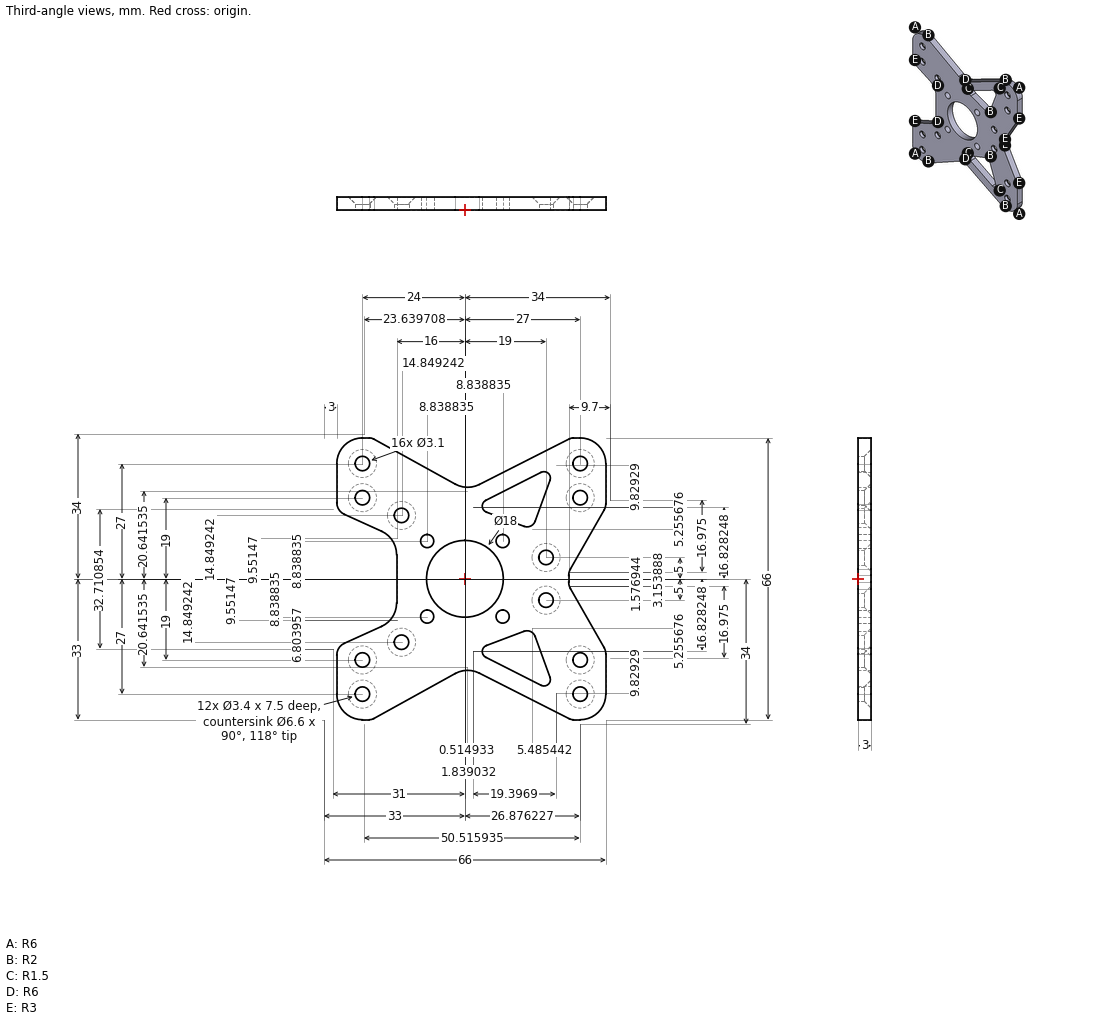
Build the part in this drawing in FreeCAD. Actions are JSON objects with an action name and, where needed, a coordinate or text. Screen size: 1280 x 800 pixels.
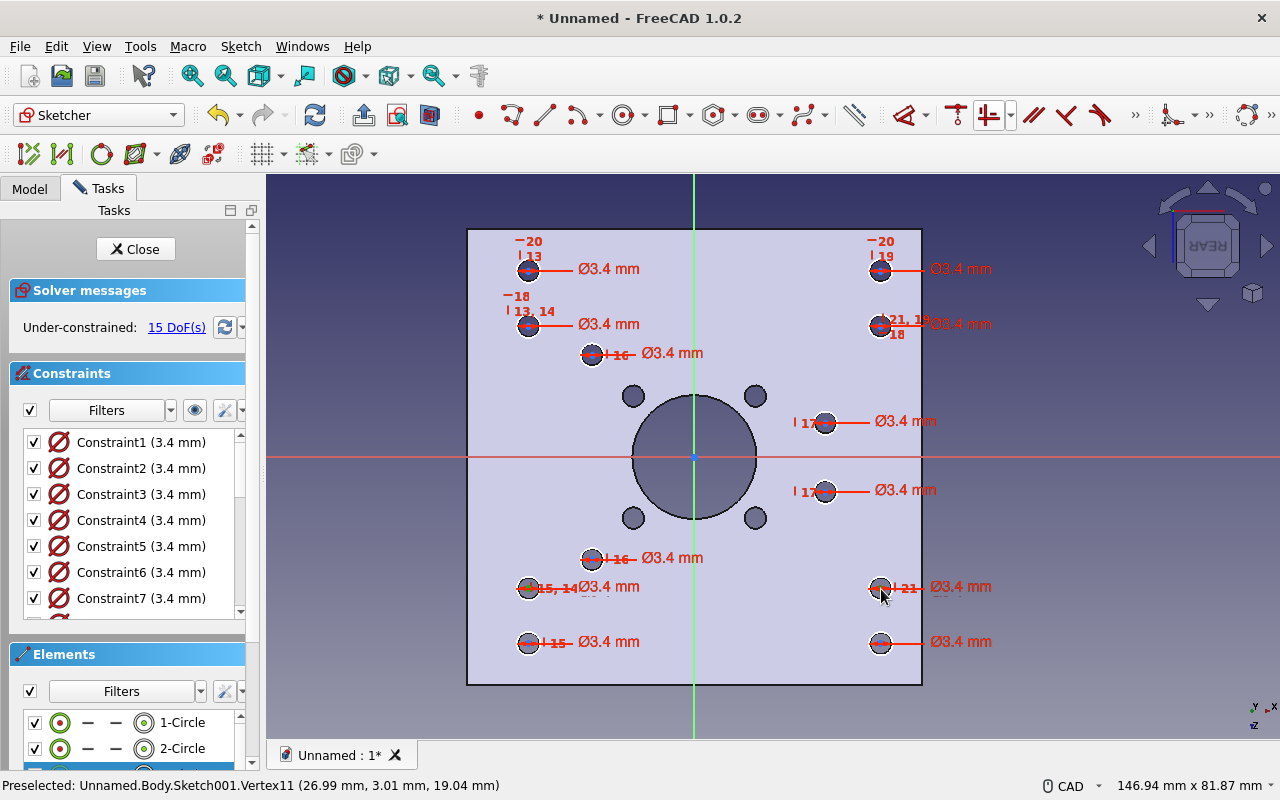
{"action": "left_click", "coordinate": [1010, 116]}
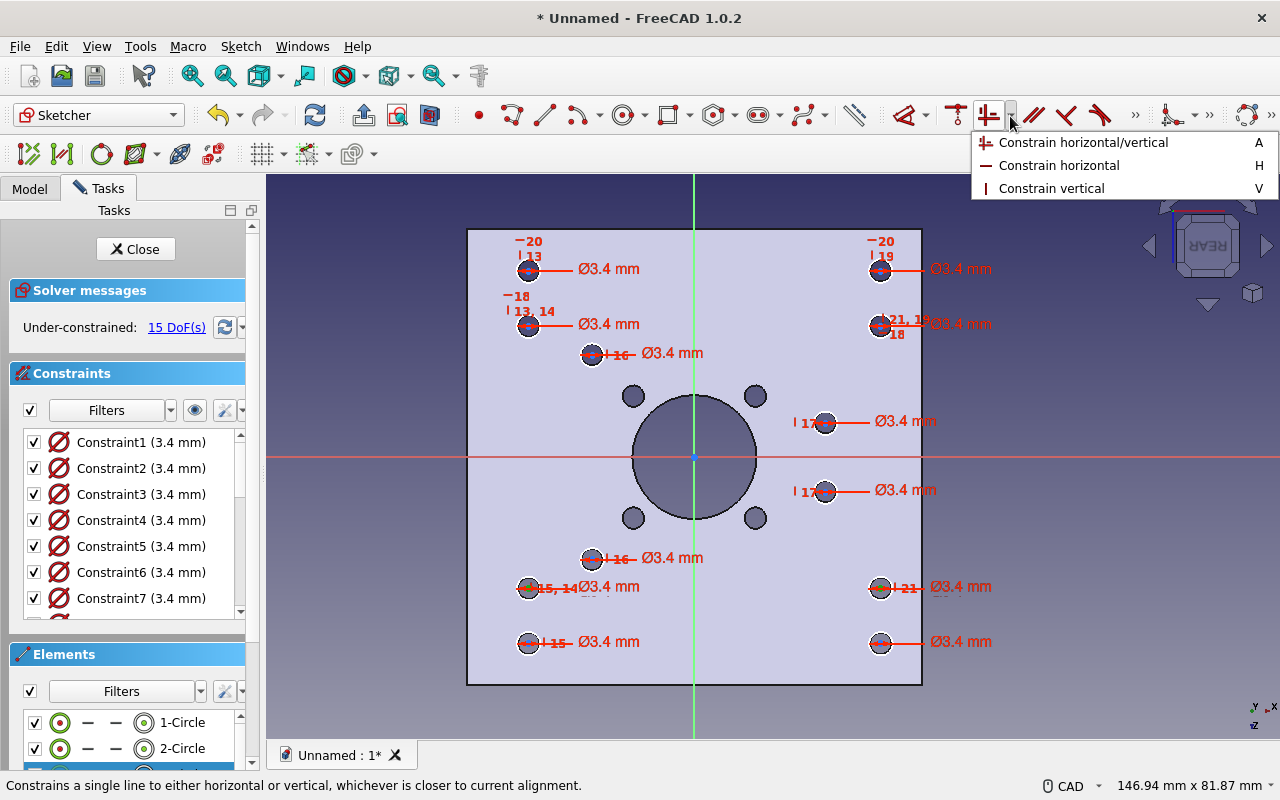
{"action": "left_click", "coordinate": [1125, 166]}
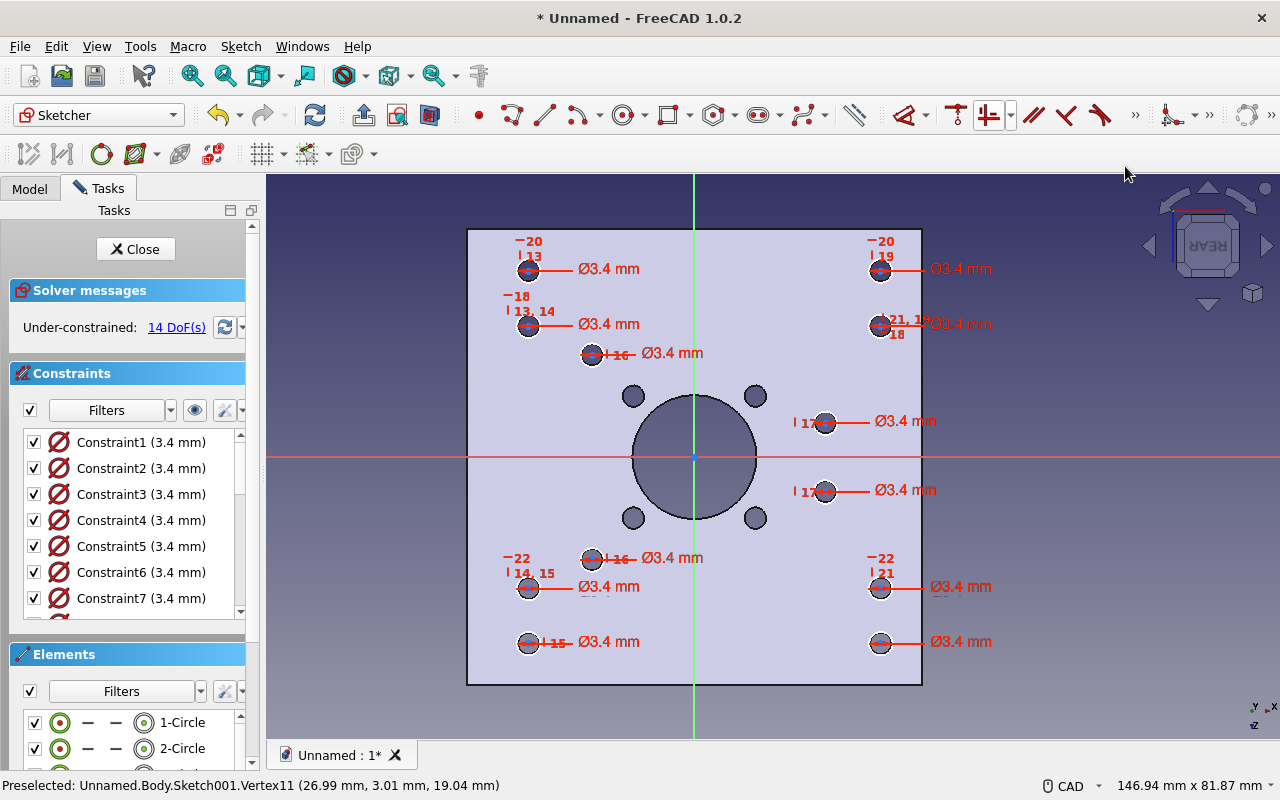
{"action": "left_click", "coordinate": [881, 589]}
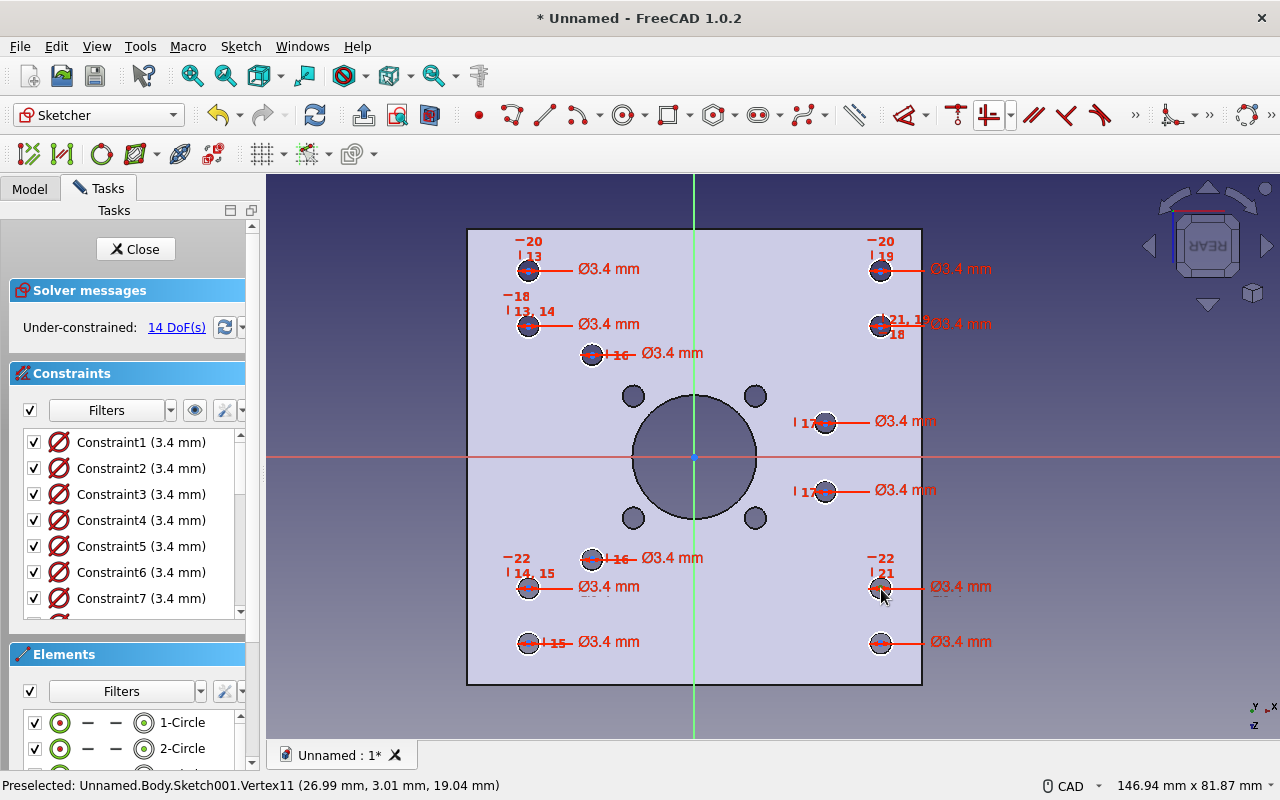
{"action": "left_click", "coordinate": [881, 644]}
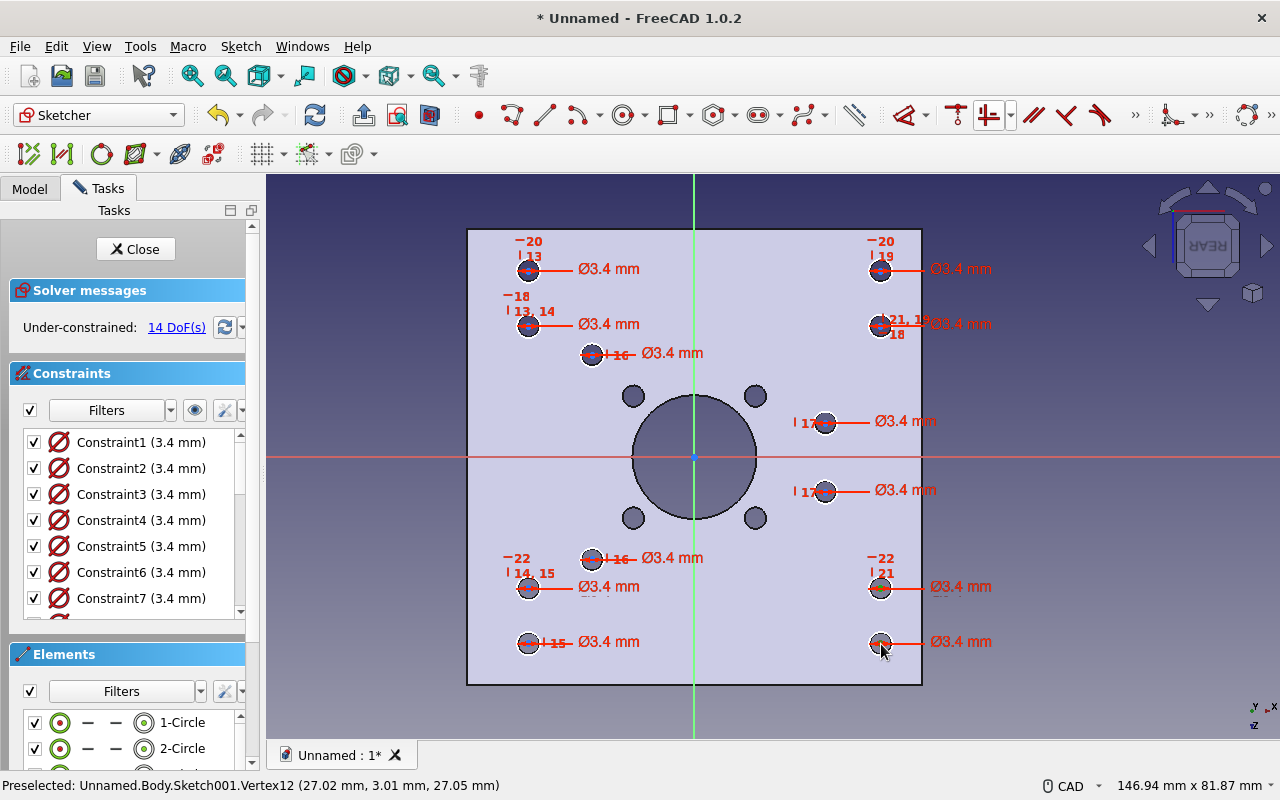
{"action": "key", "text": "v"}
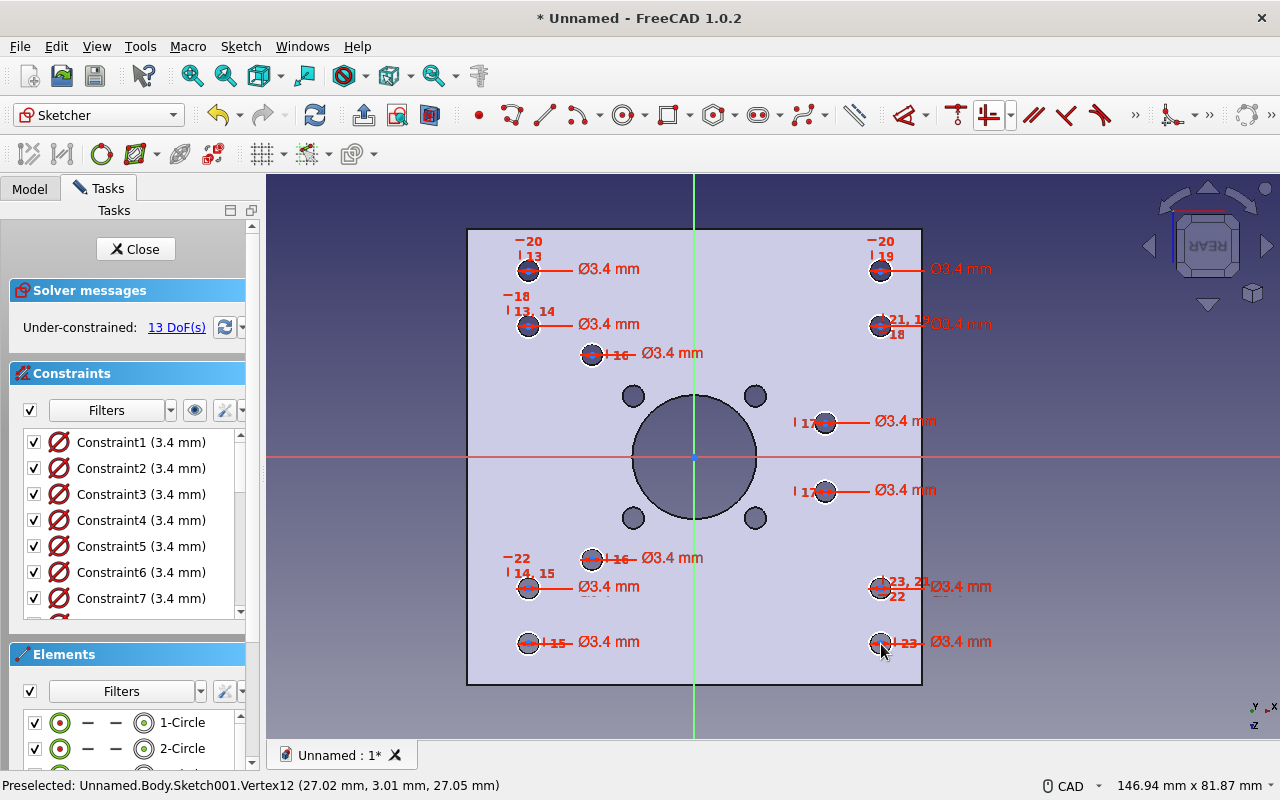
{"action": "left_click", "coordinate": [529, 644]}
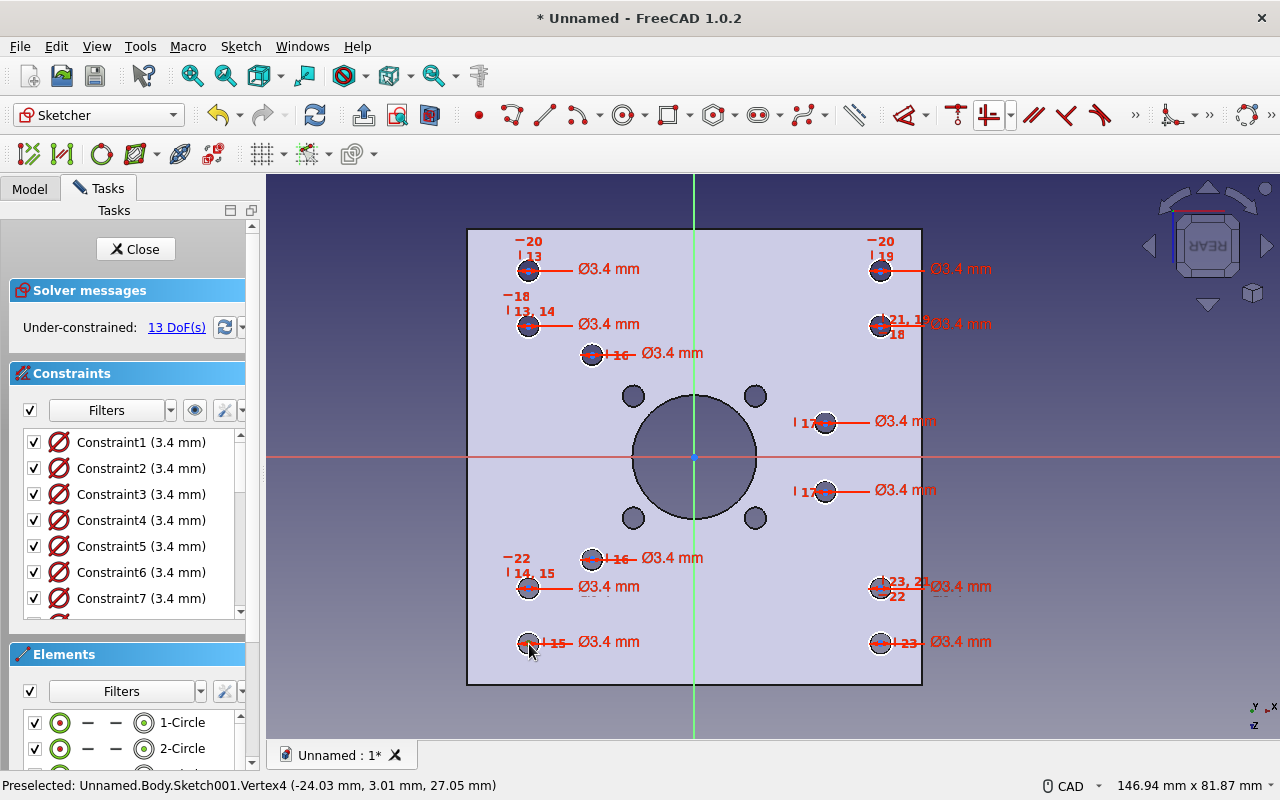
{"action": "left_click", "coordinate": [881, 644]}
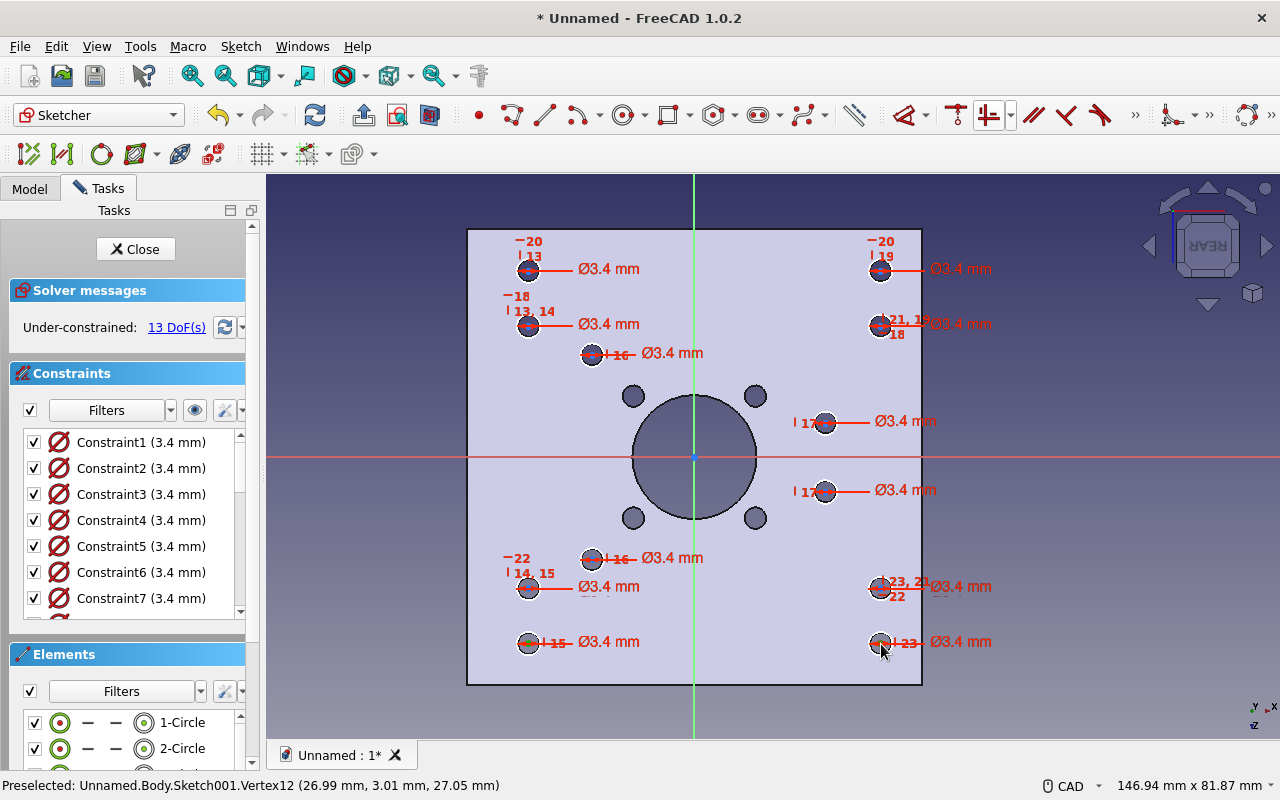
{"action": "key", "text": "h"}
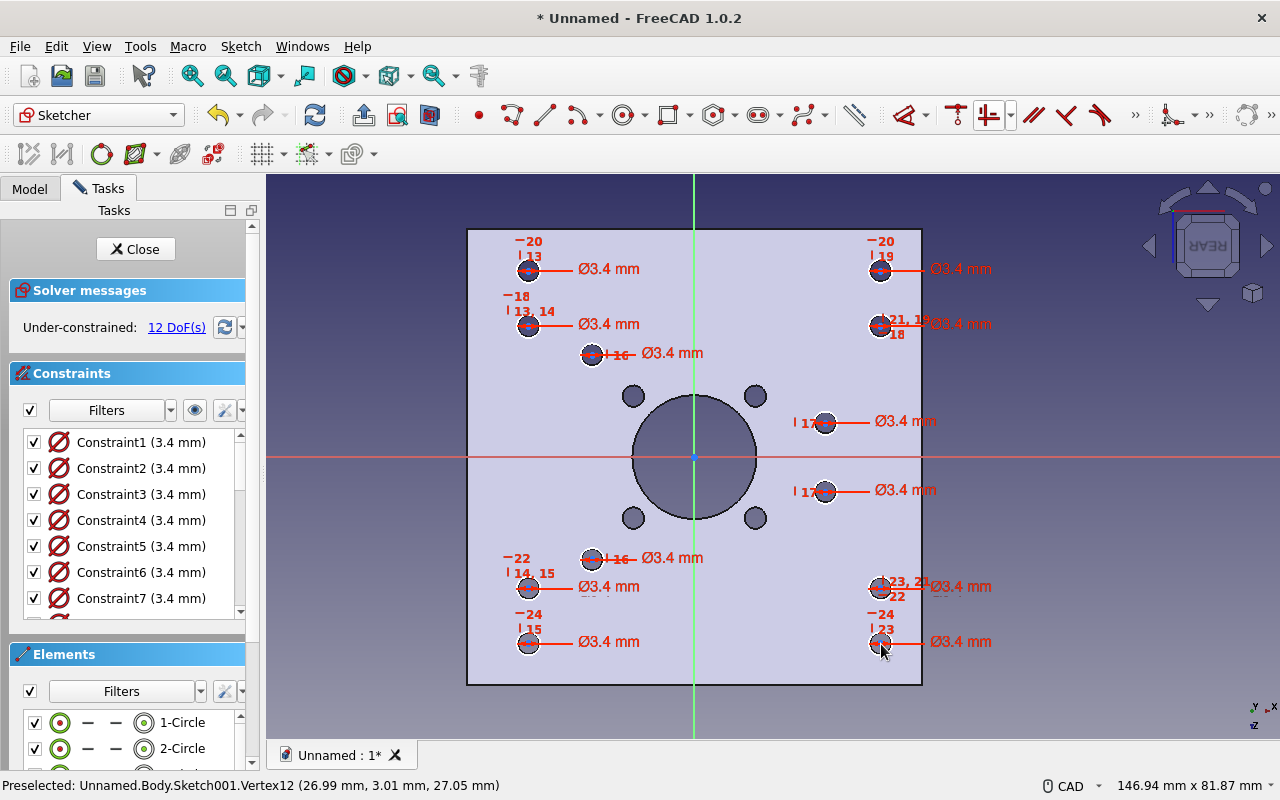
{"action": "left_click", "coordinate": [904, 116]}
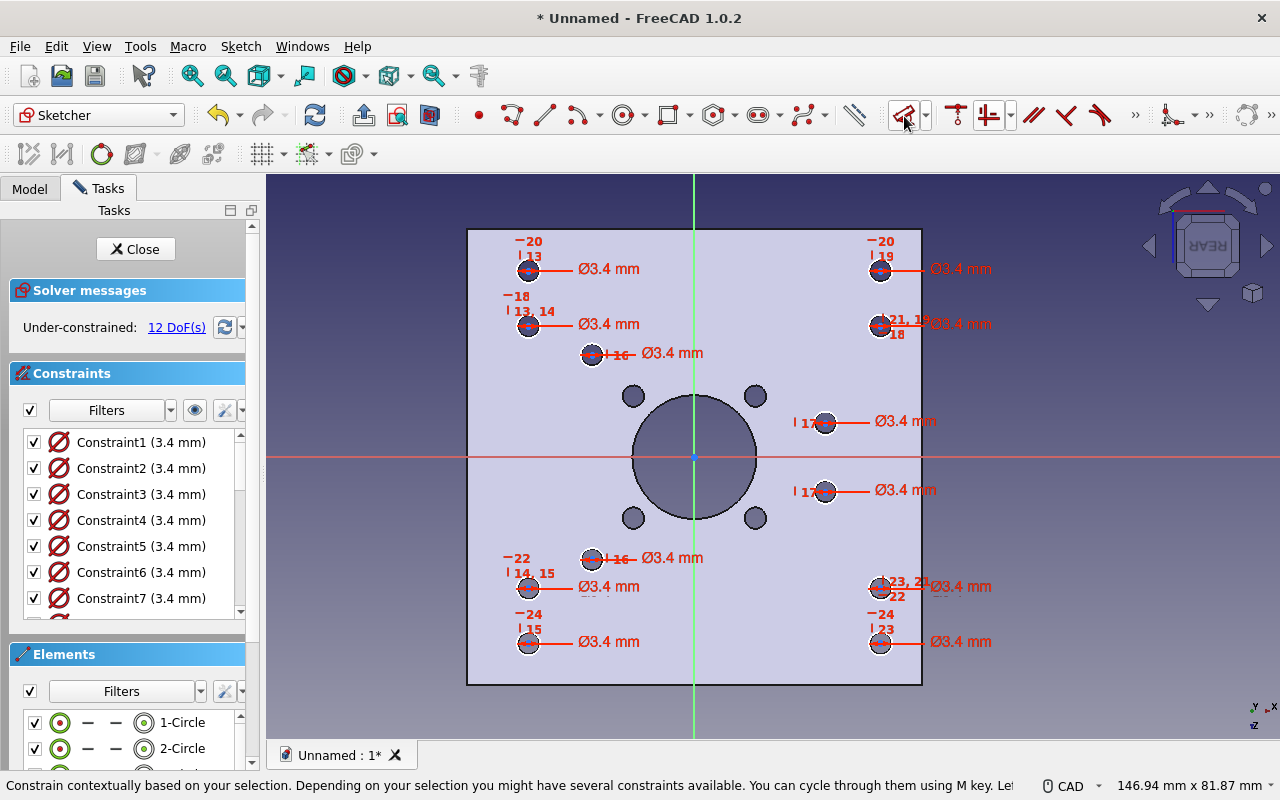
{"action": "left_click", "coordinate": [825, 492]}
{"action": "left_click", "coordinate": [859, 475]}